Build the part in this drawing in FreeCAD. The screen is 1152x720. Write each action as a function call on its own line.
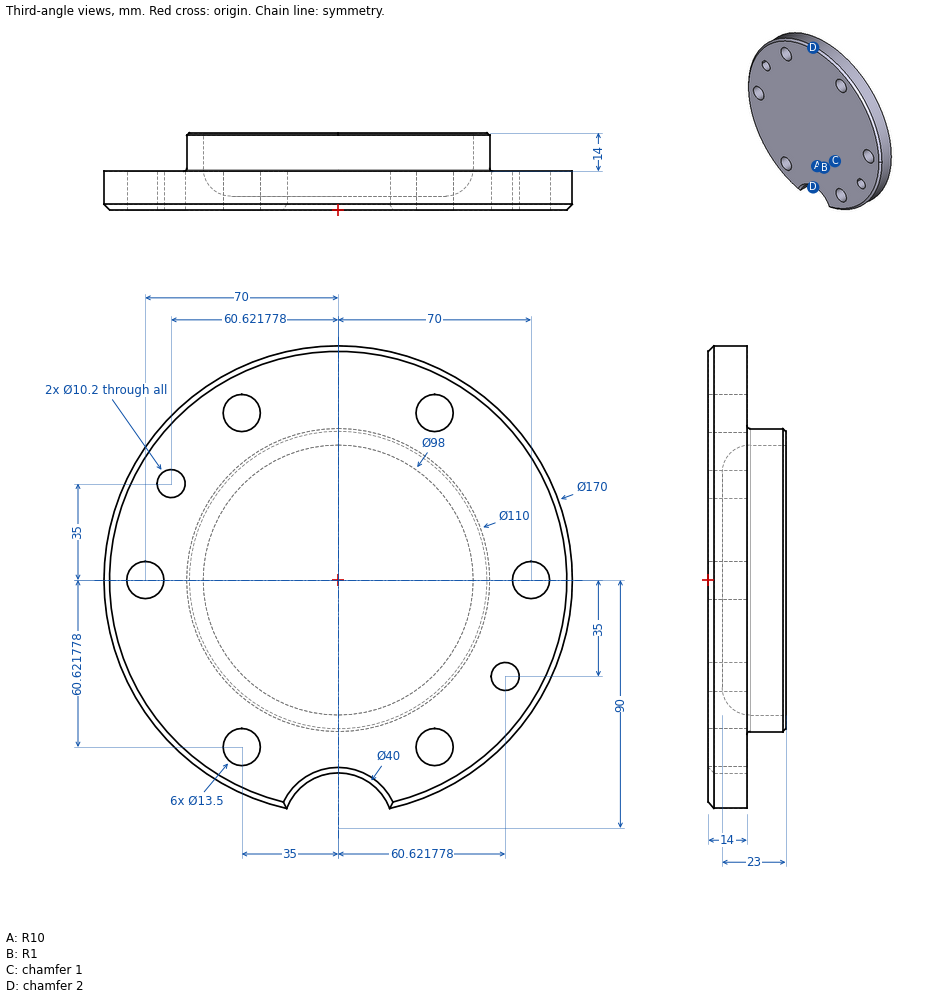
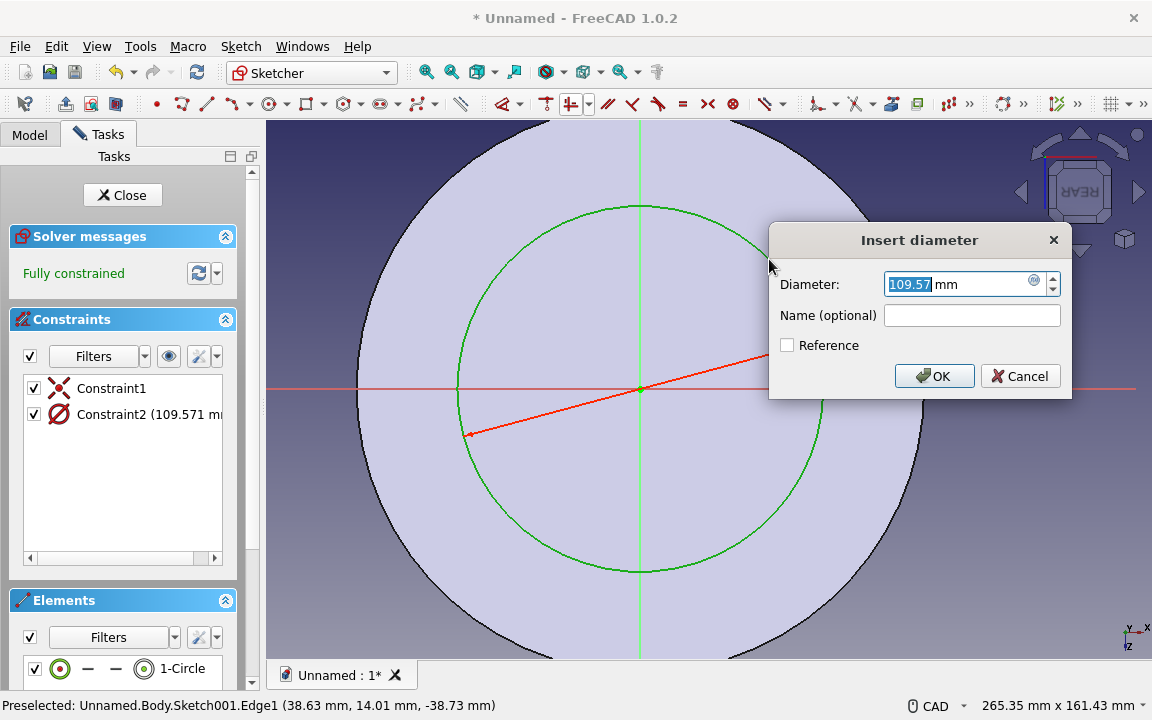
text(110)
key(Return)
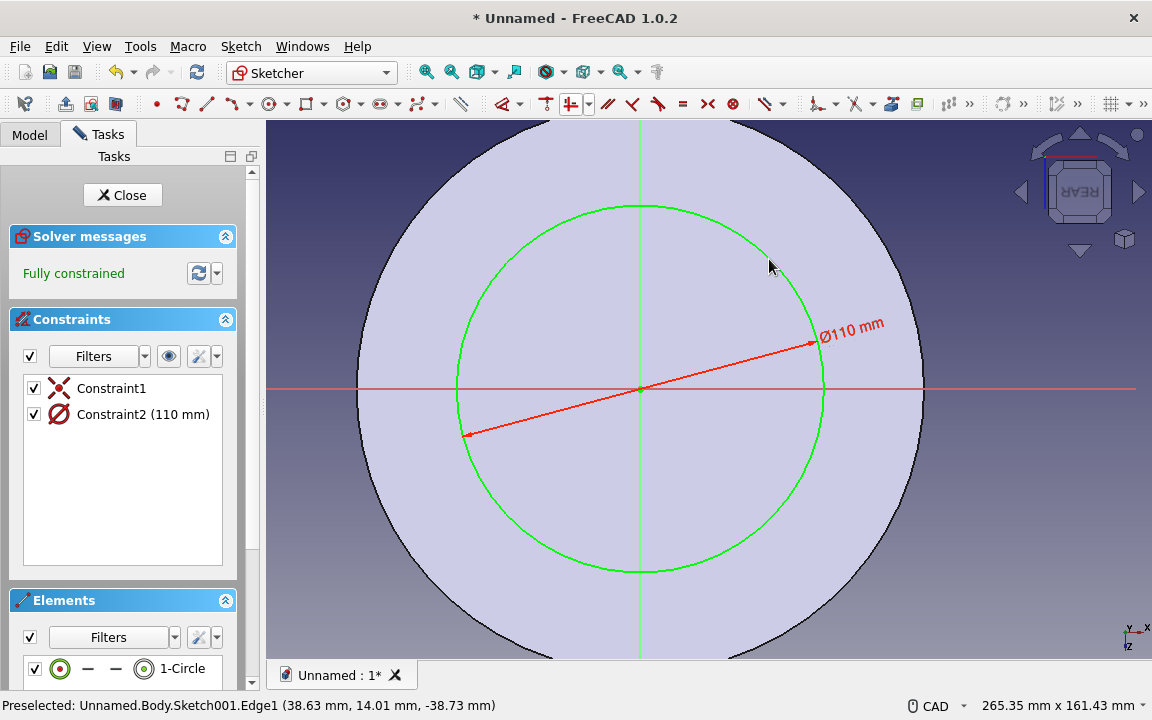
click(123, 195)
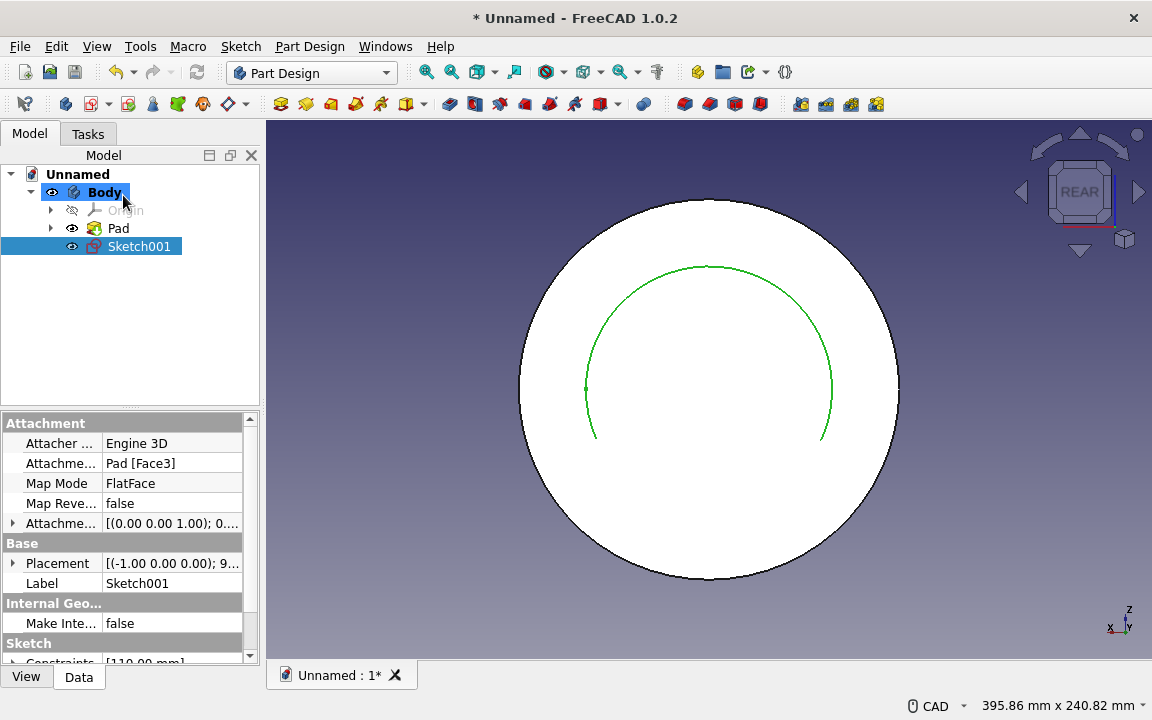
click(281, 104)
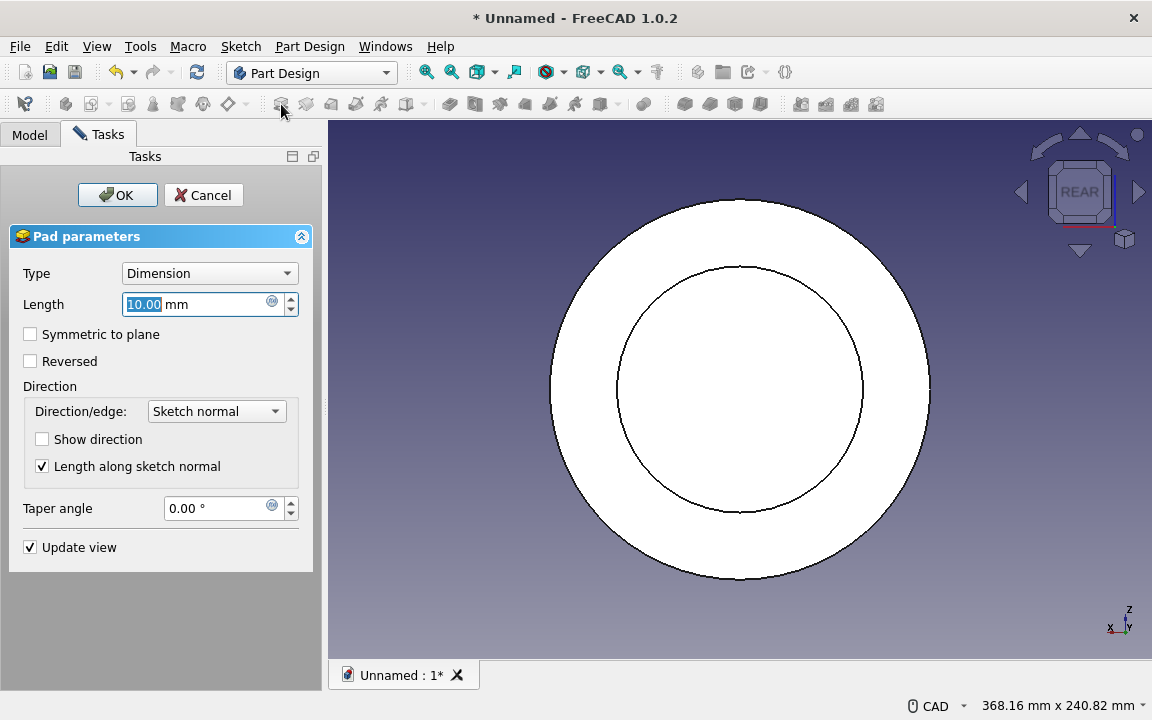
text(14)
key(Tab)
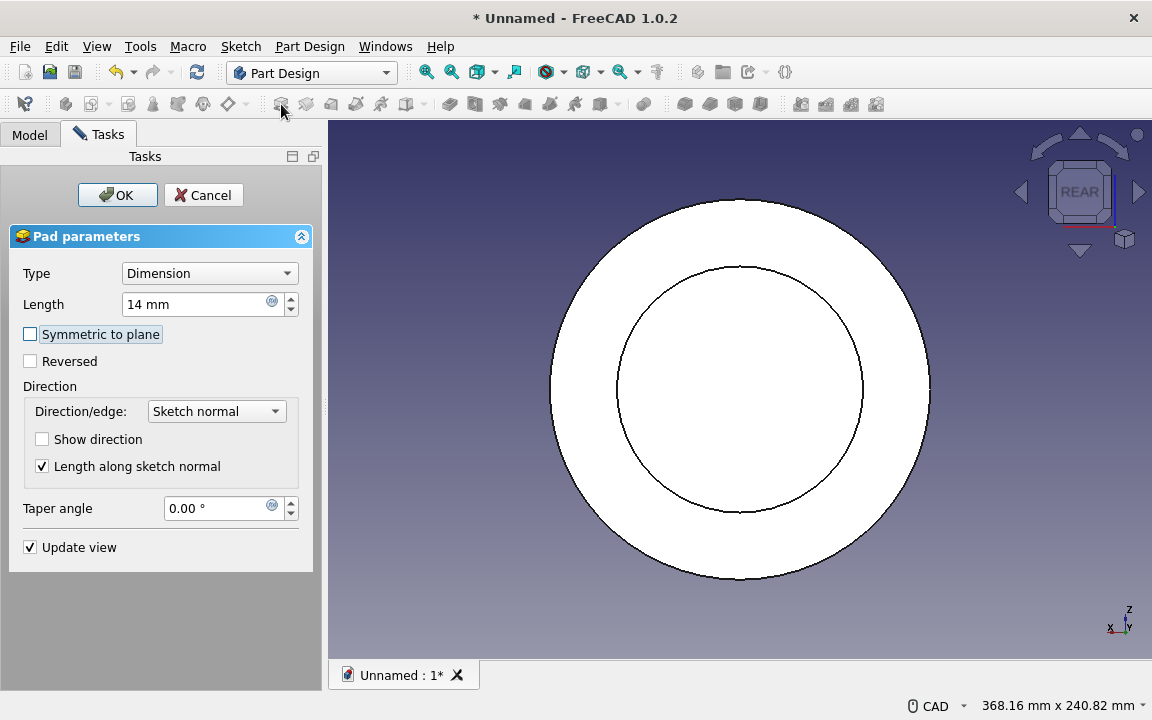
click(118, 195)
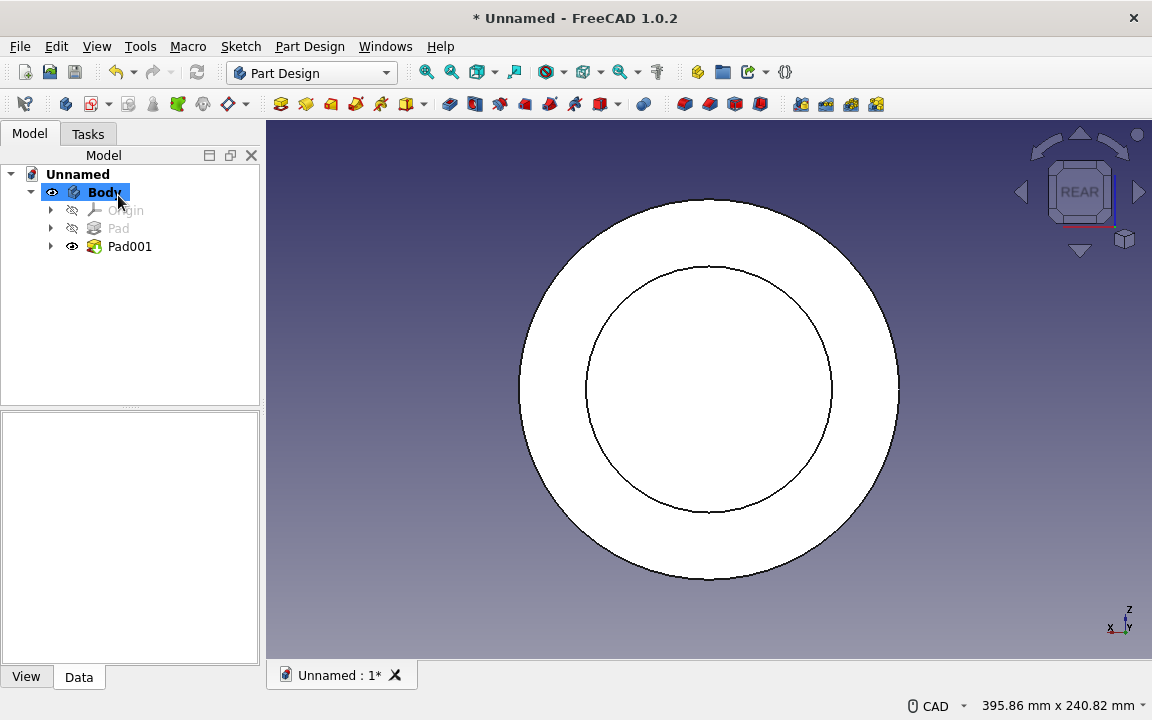
click(709, 388)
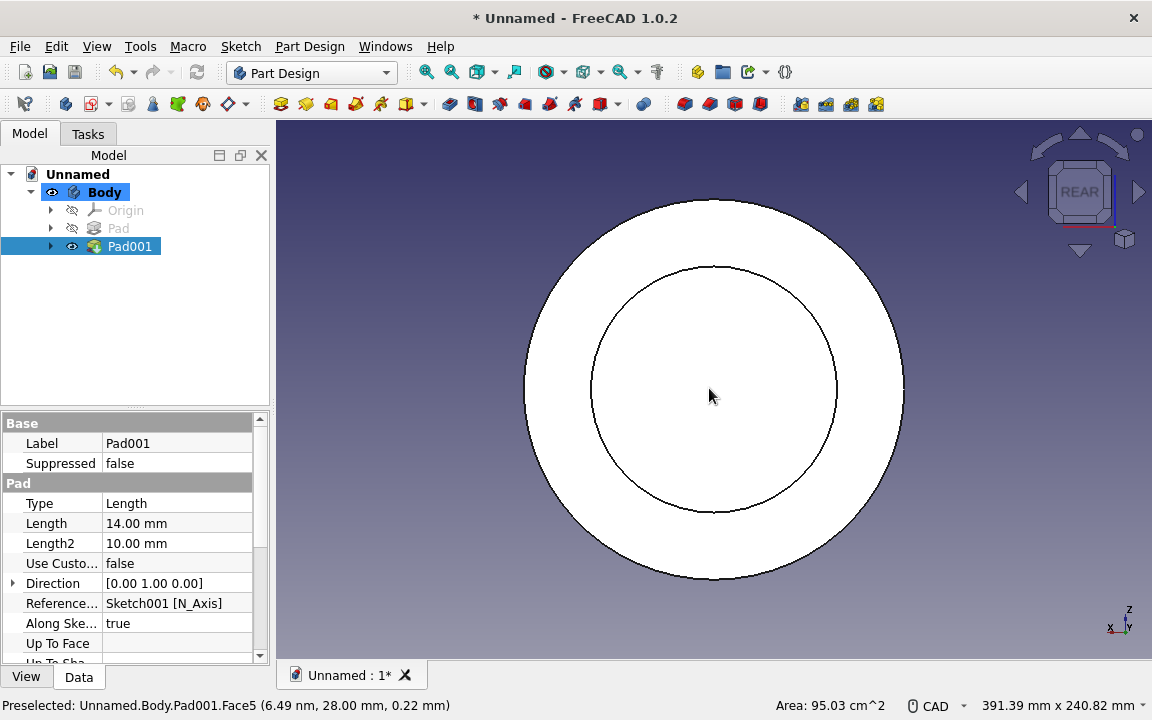
click(90, 104)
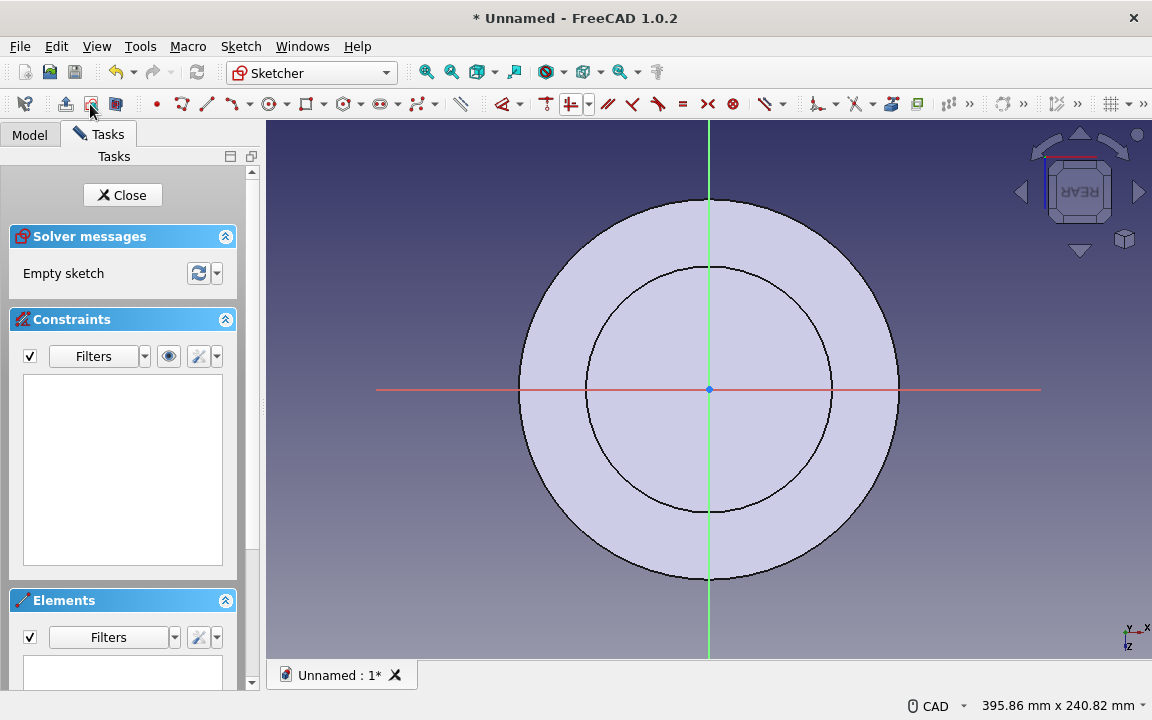
scroll(848, 389, up, 2)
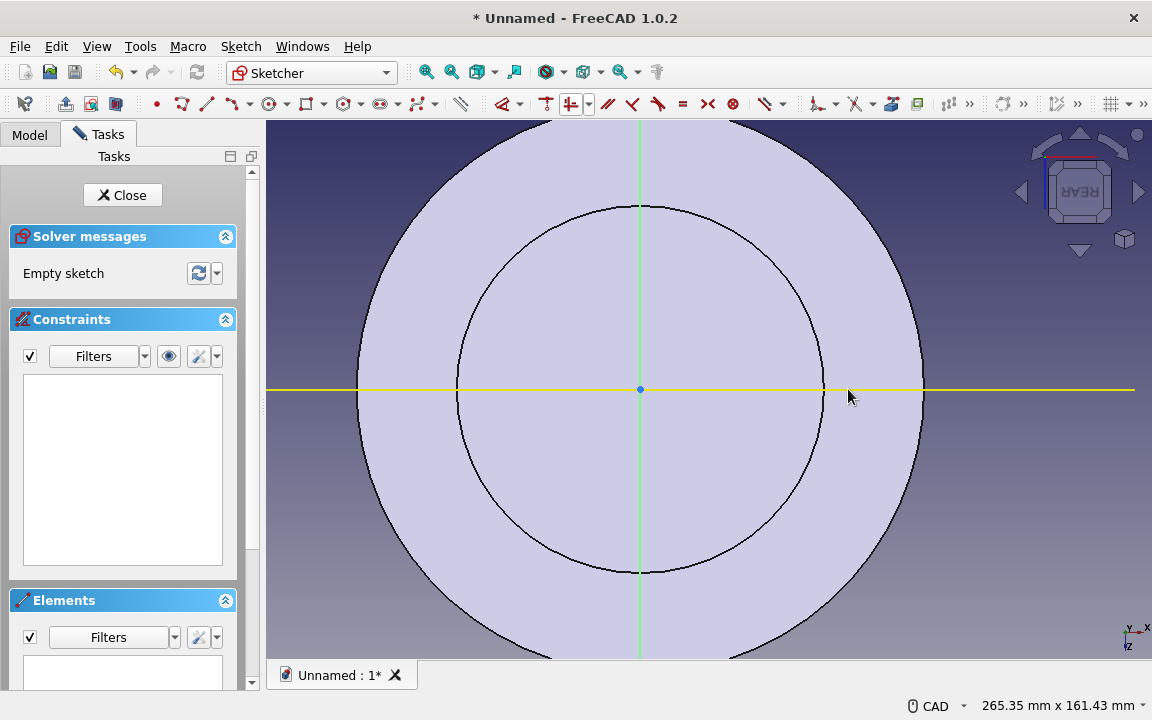
click(268, 104)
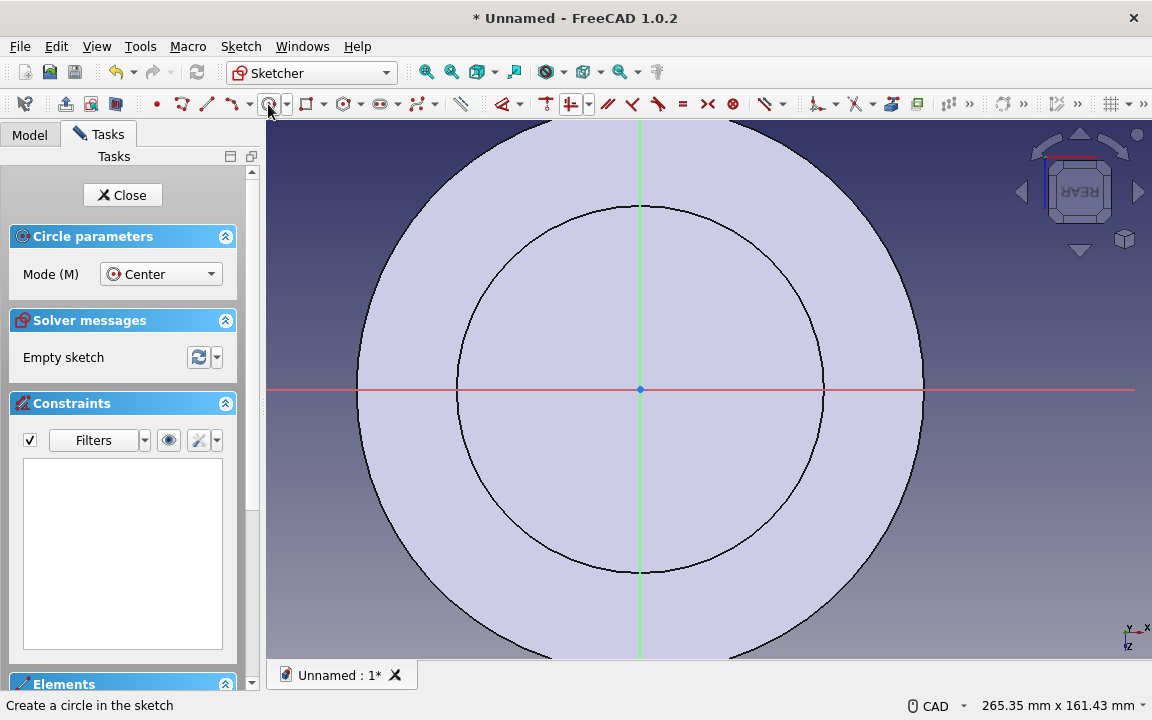
click(640, 389)
click(756, 274)
key(Escape)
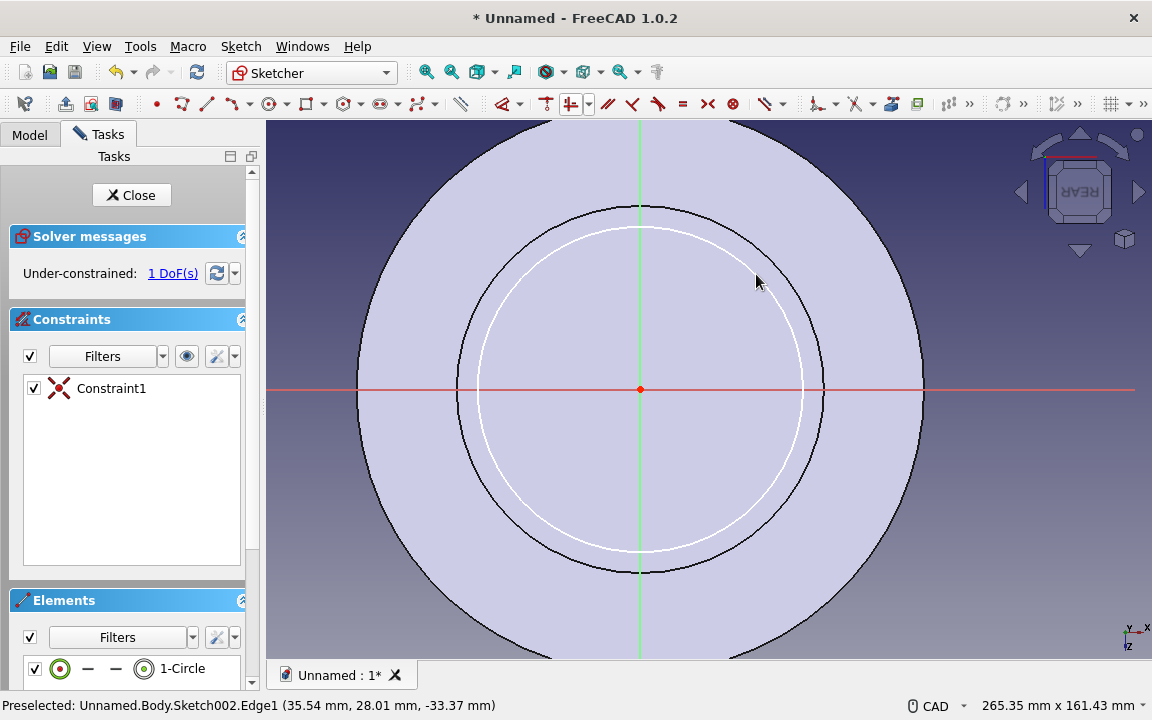
click(755, 274)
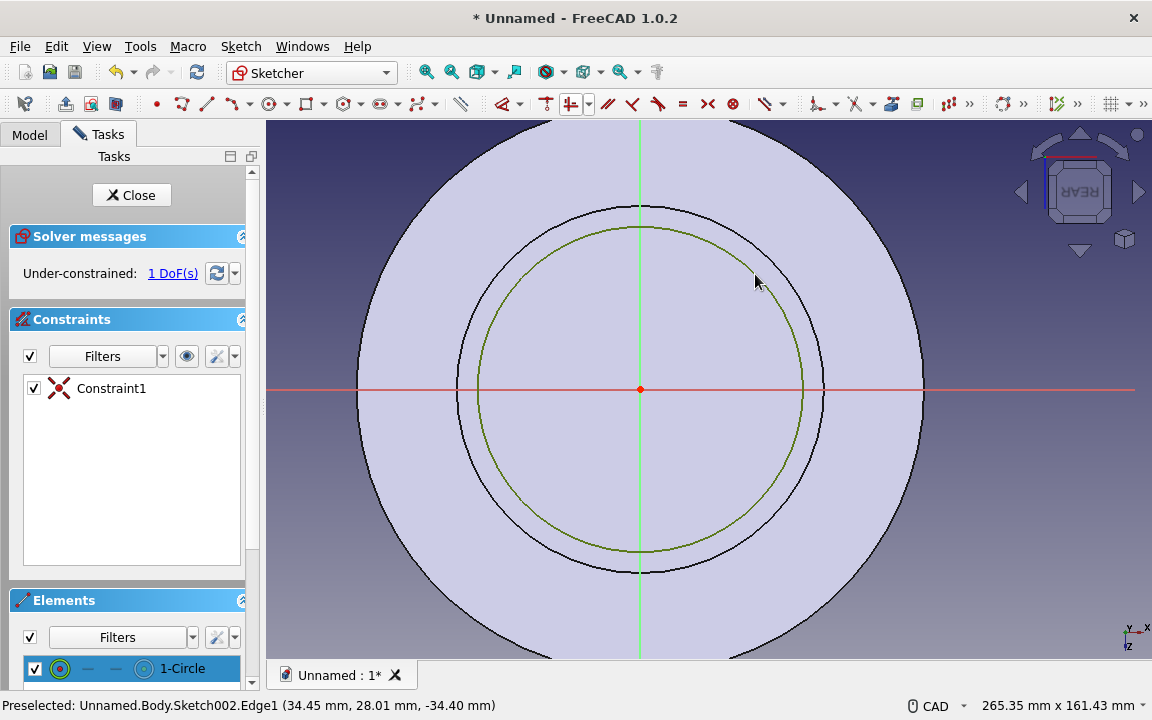
click(520, 104)